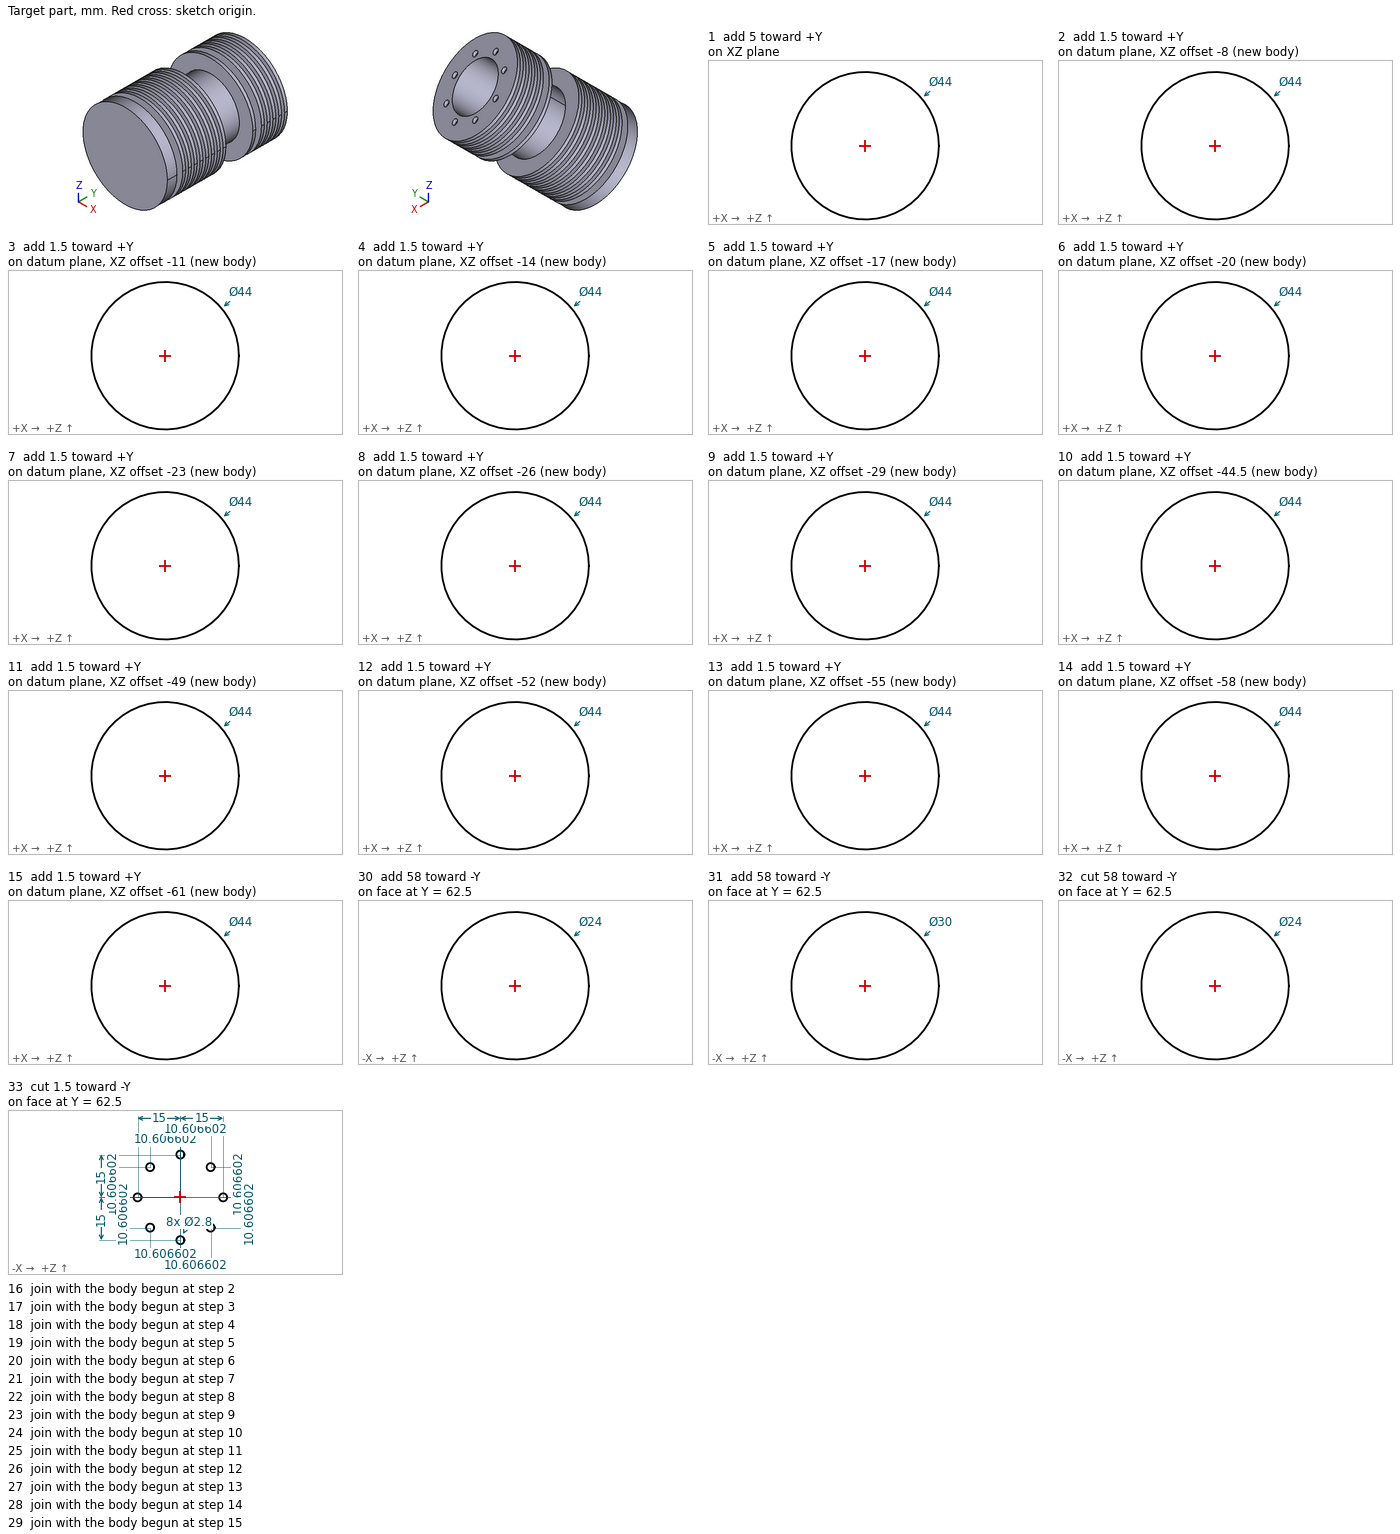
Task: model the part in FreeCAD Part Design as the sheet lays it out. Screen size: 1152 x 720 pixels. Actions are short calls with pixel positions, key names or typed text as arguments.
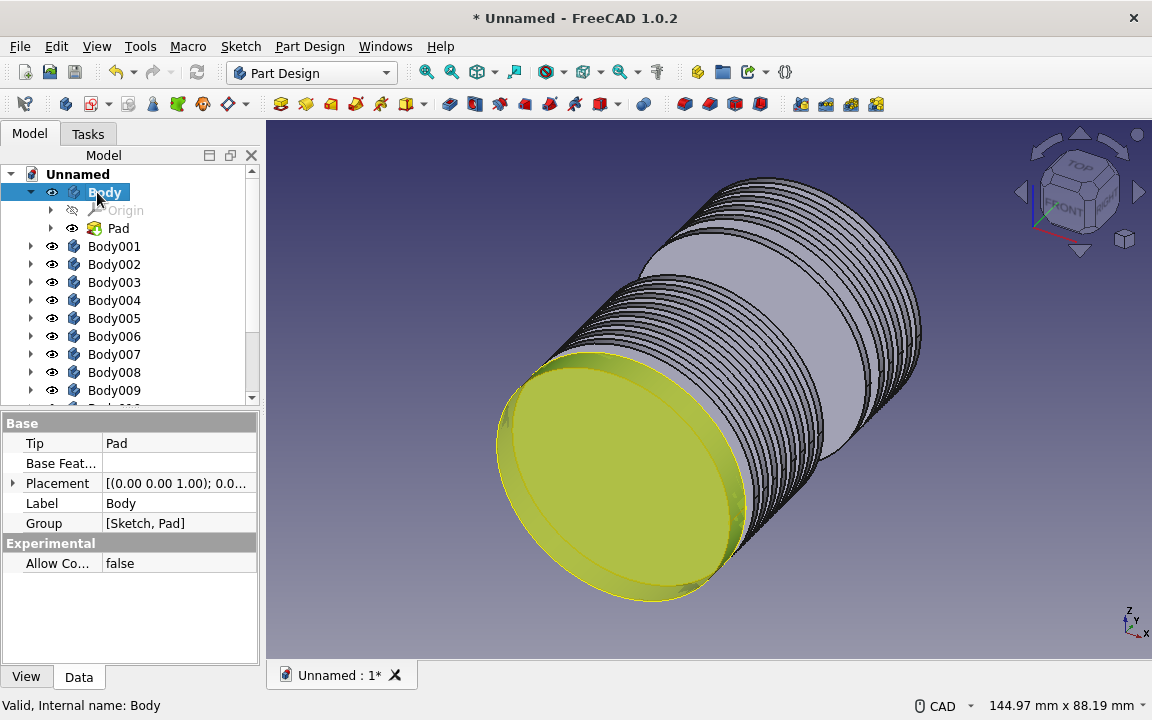
click(97, 192)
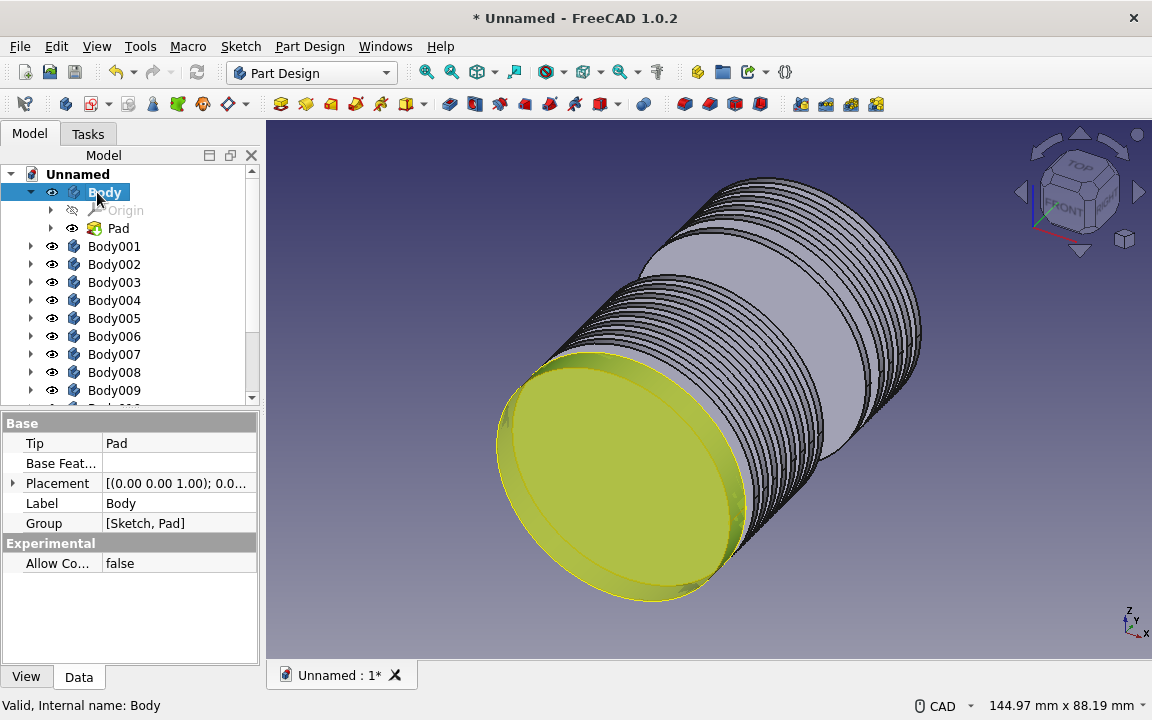
click(148, 563)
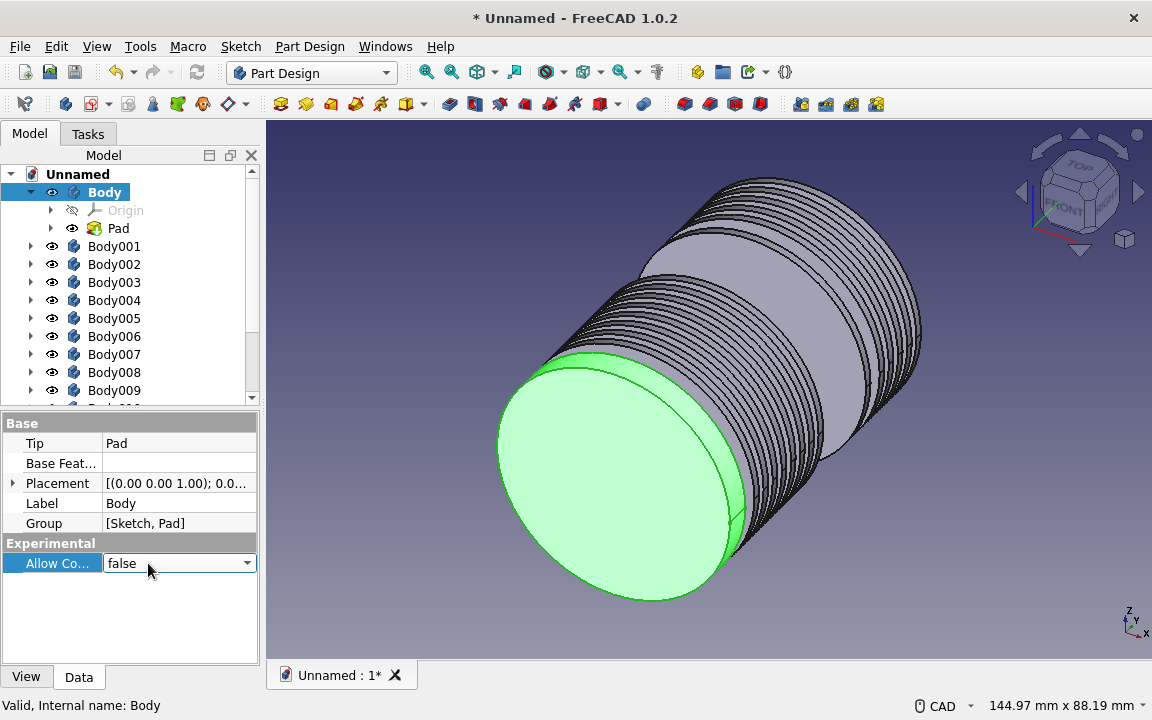
click(148, 563)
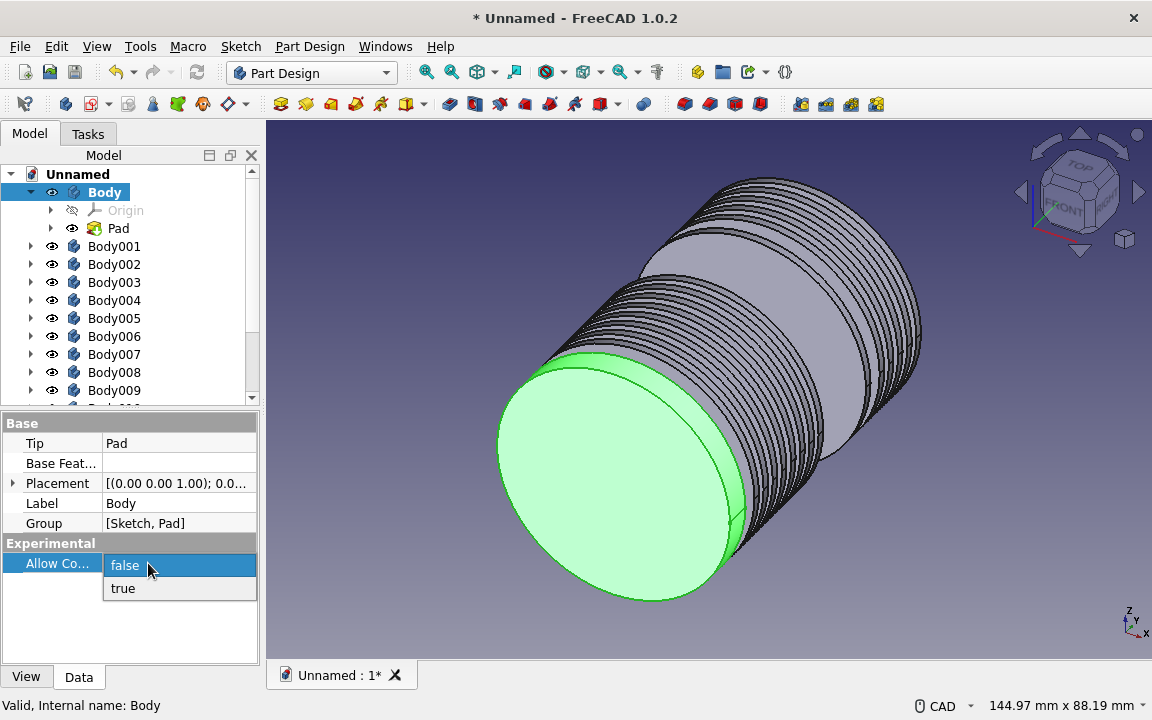
click(178, 588)
key(Return)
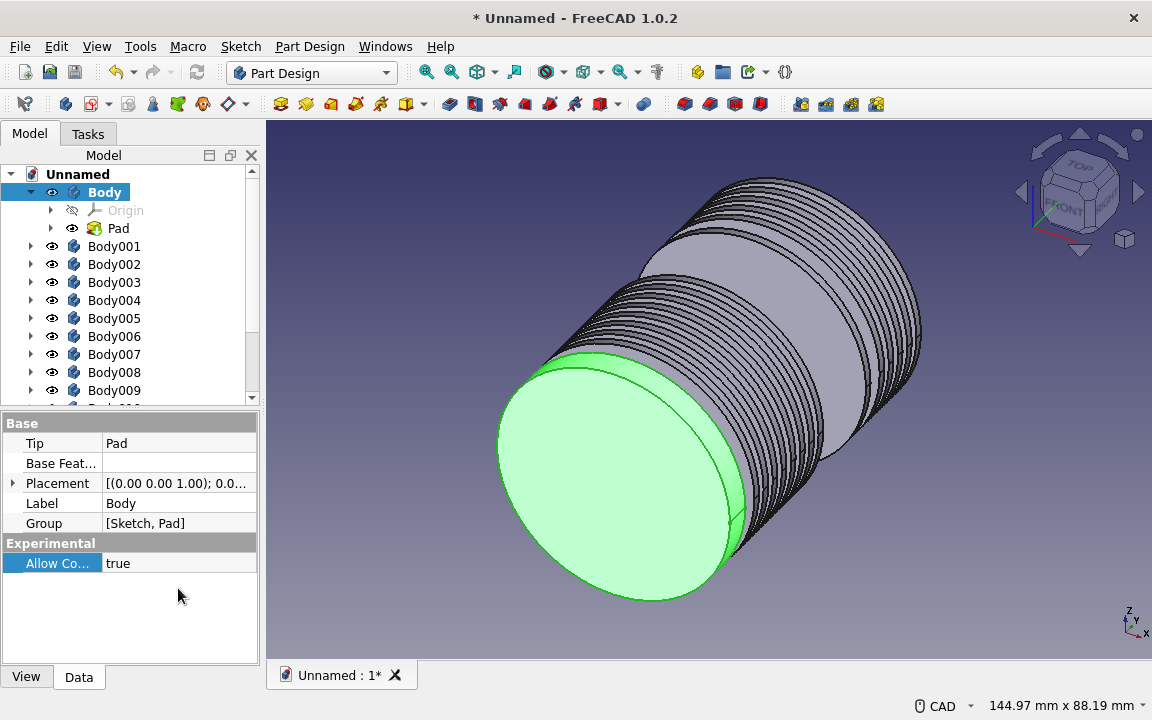
click(97, 246)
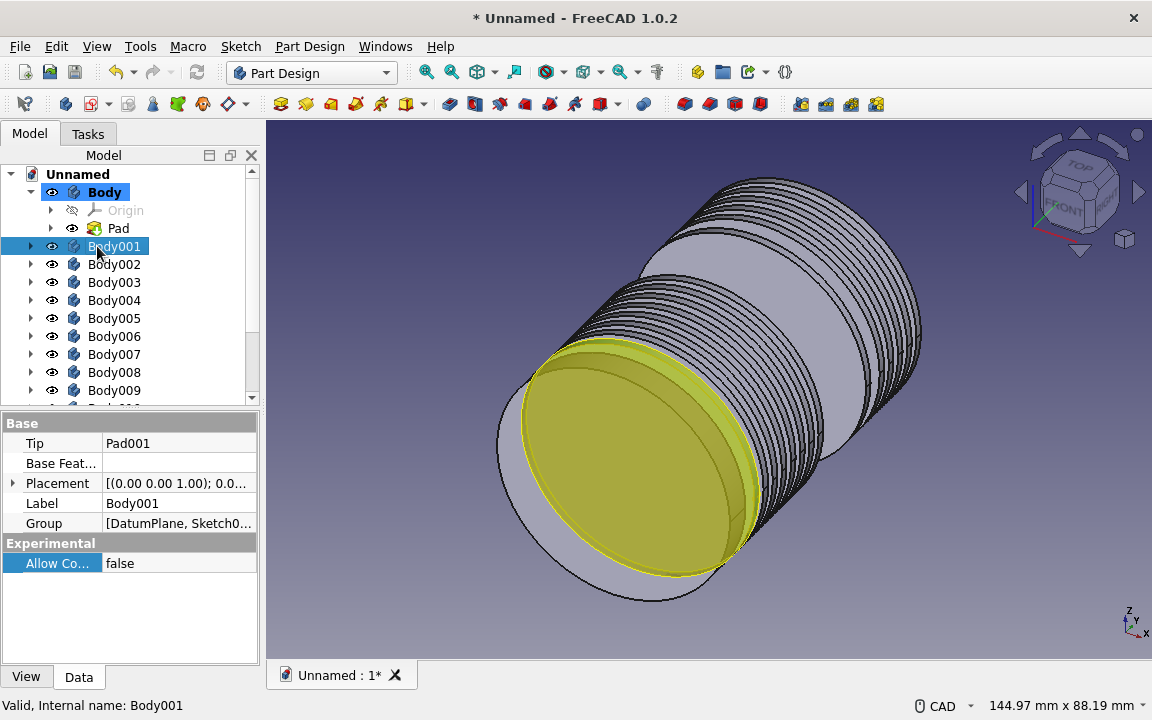
click(644, 104)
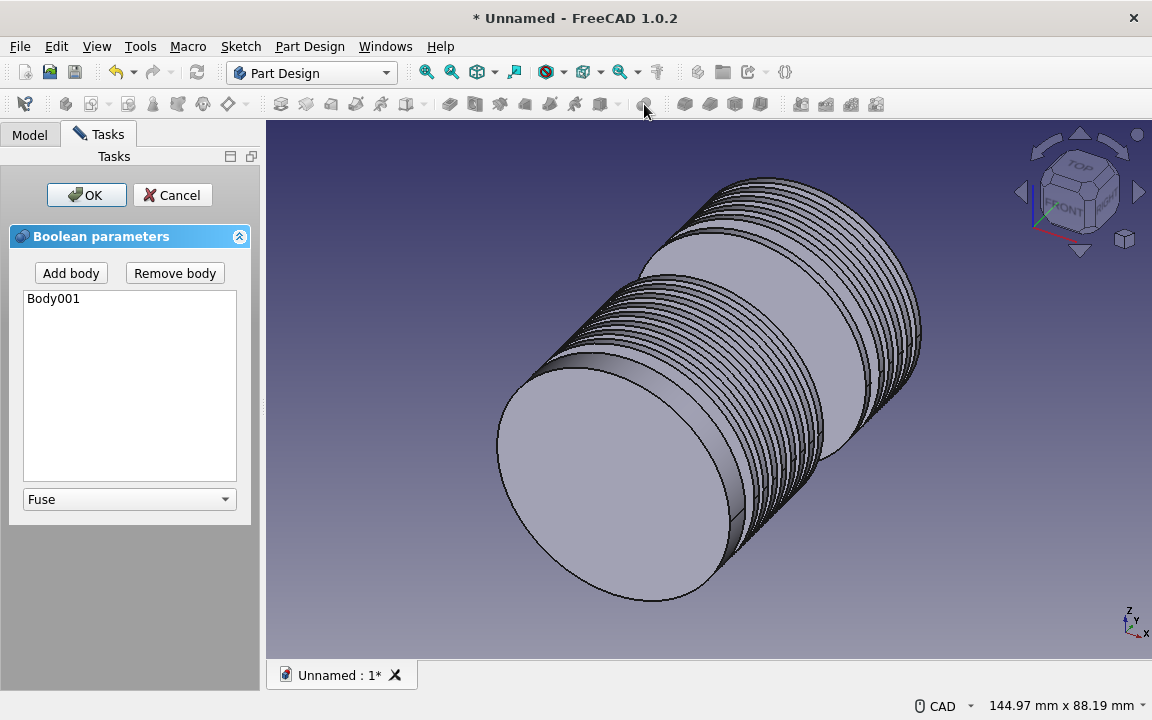
click(87, 195)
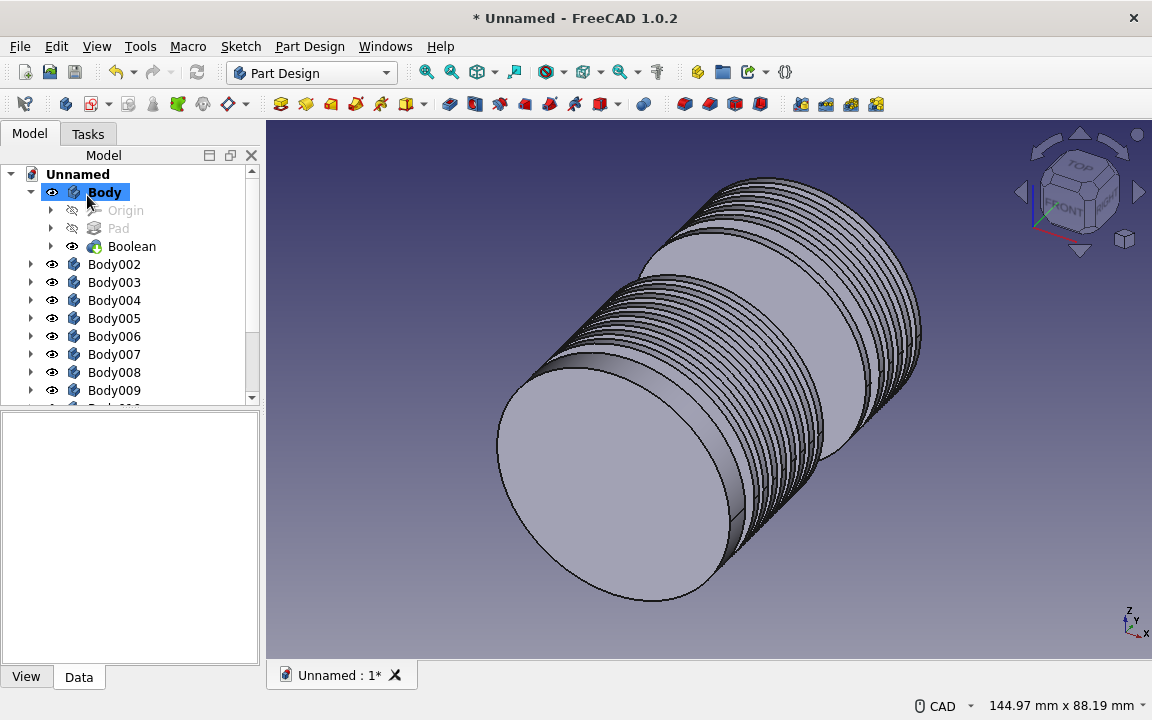
click(97, 264)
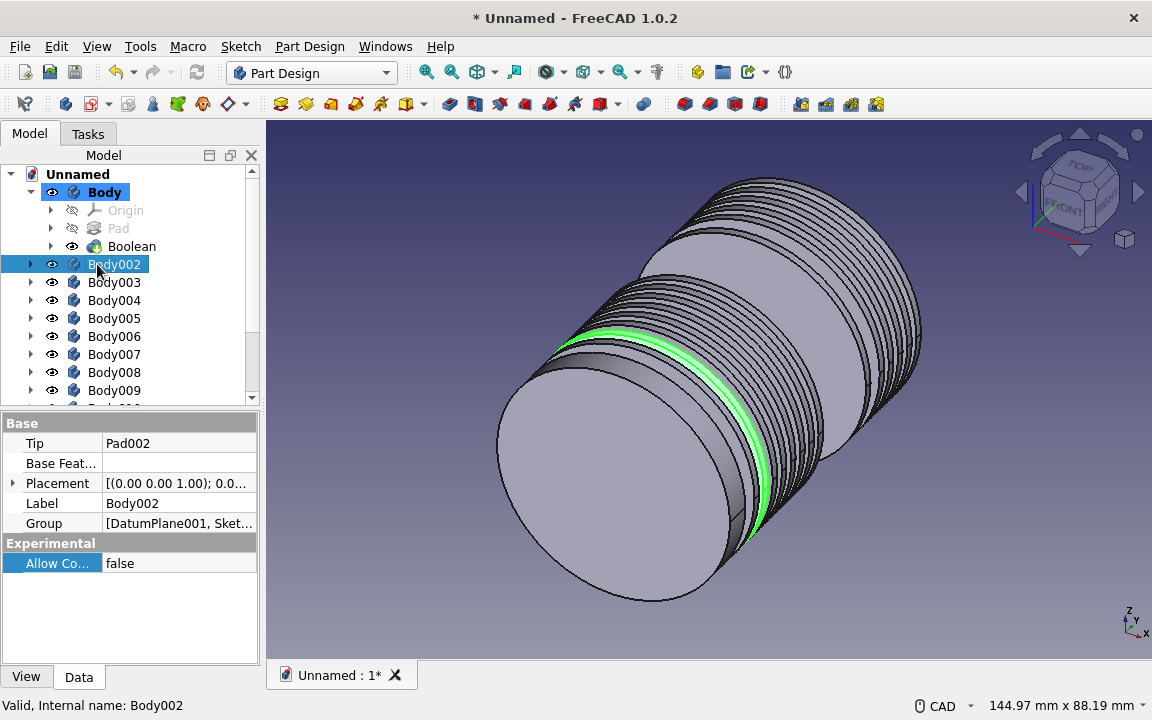
click(644, 104)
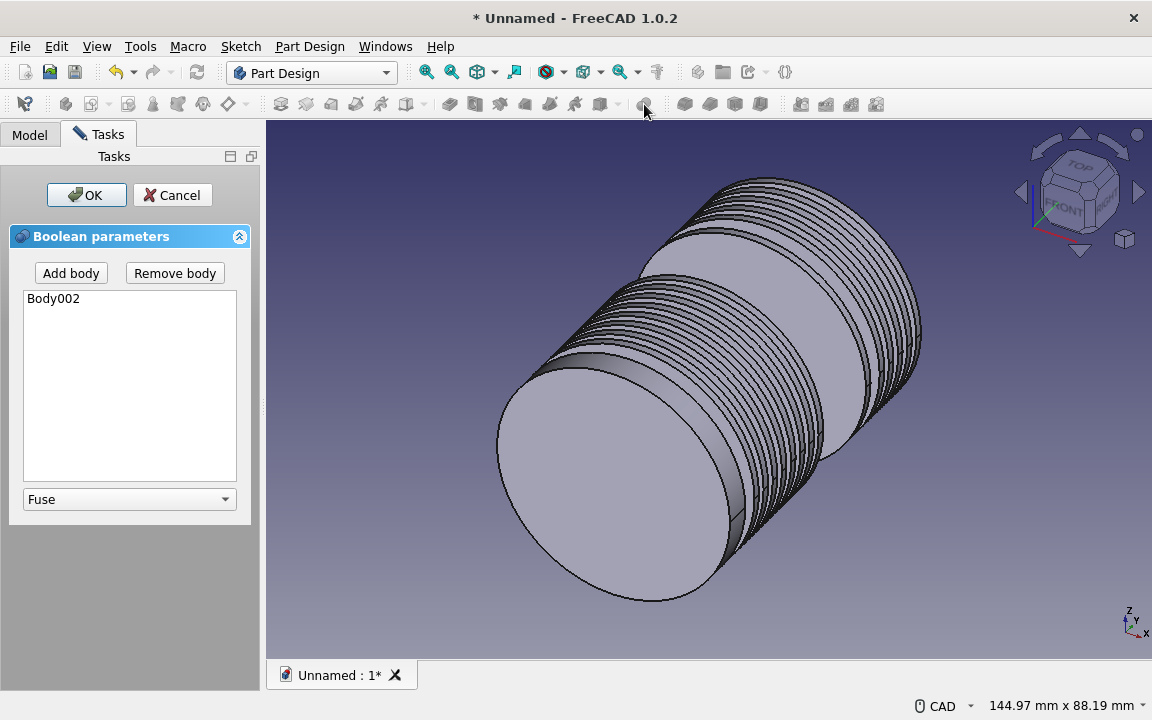
click(87, 195)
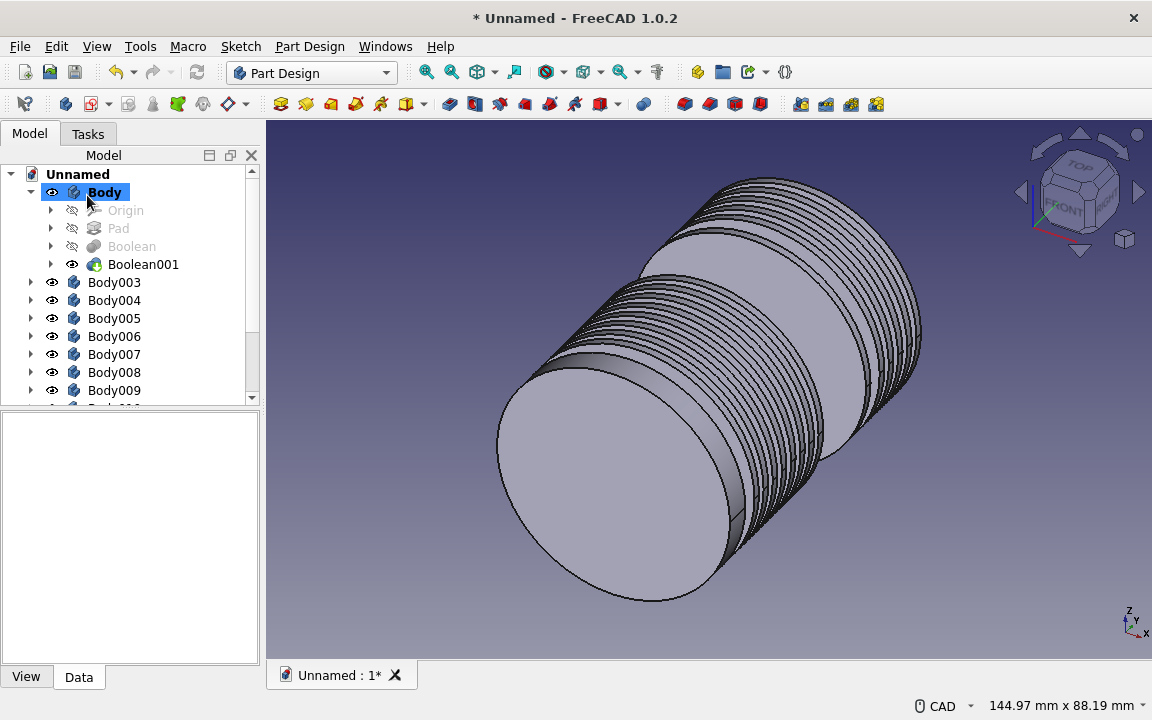
click(97, 282)